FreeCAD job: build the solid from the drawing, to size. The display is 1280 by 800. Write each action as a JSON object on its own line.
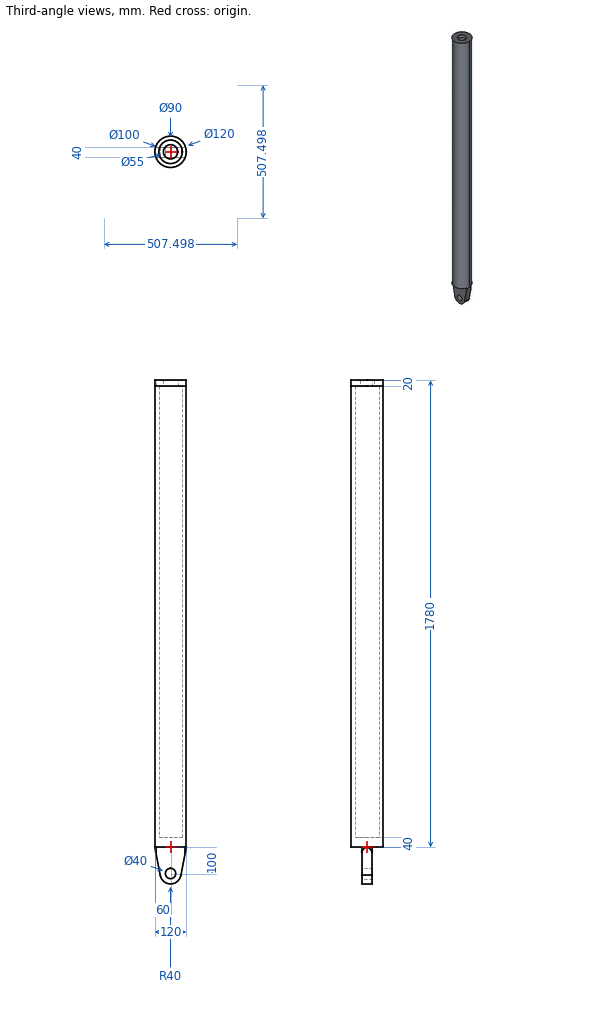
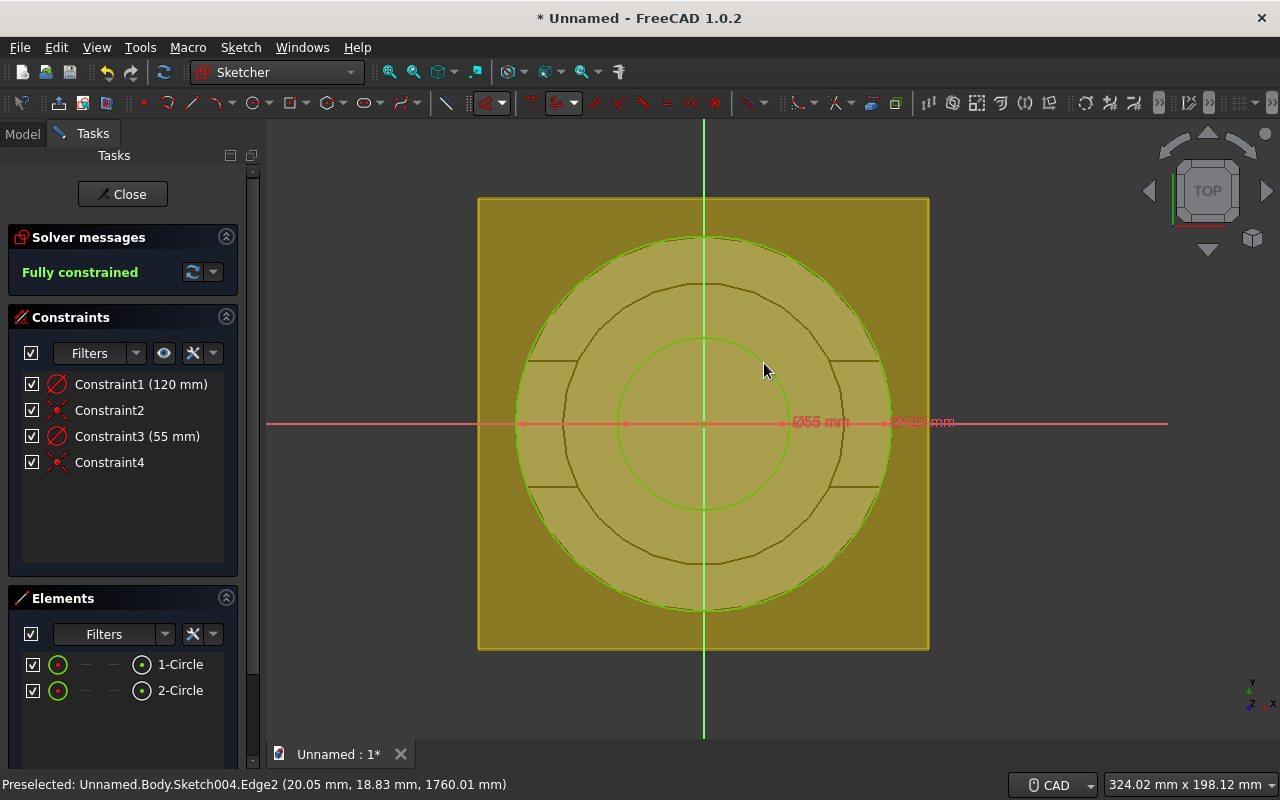
{"action": "left_click", "coordinate": [123, 194]}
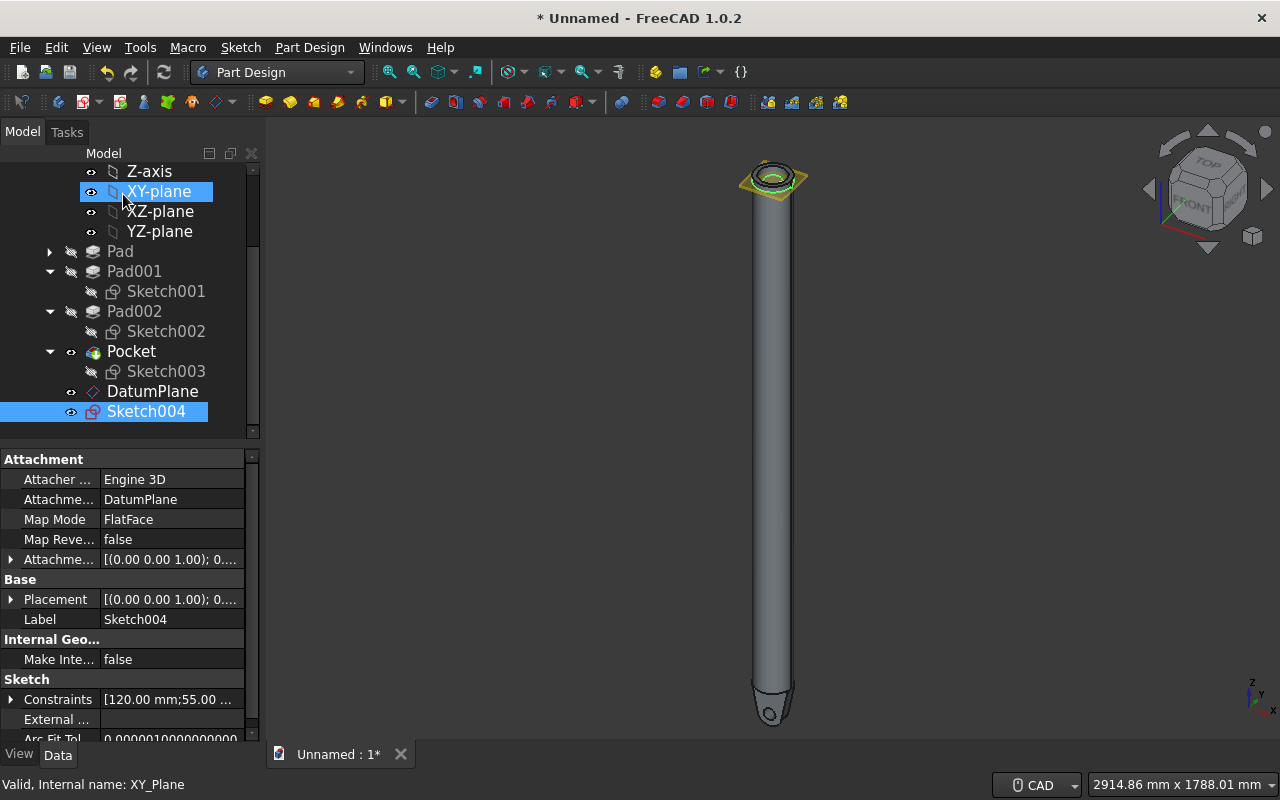
{"action": "left_click", "coordinate": [266, 102]}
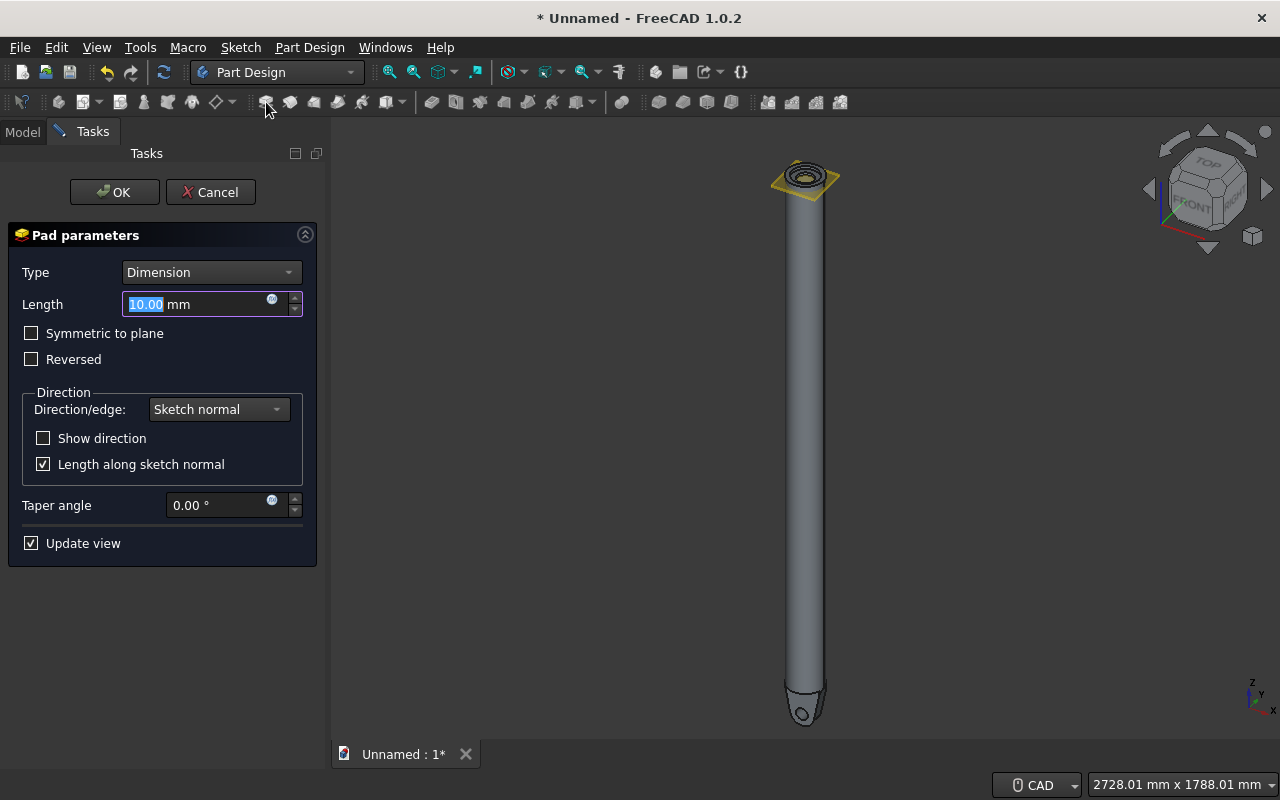
{"action": "type", "text": "20"}
{"action": "key", "text": "Tab"}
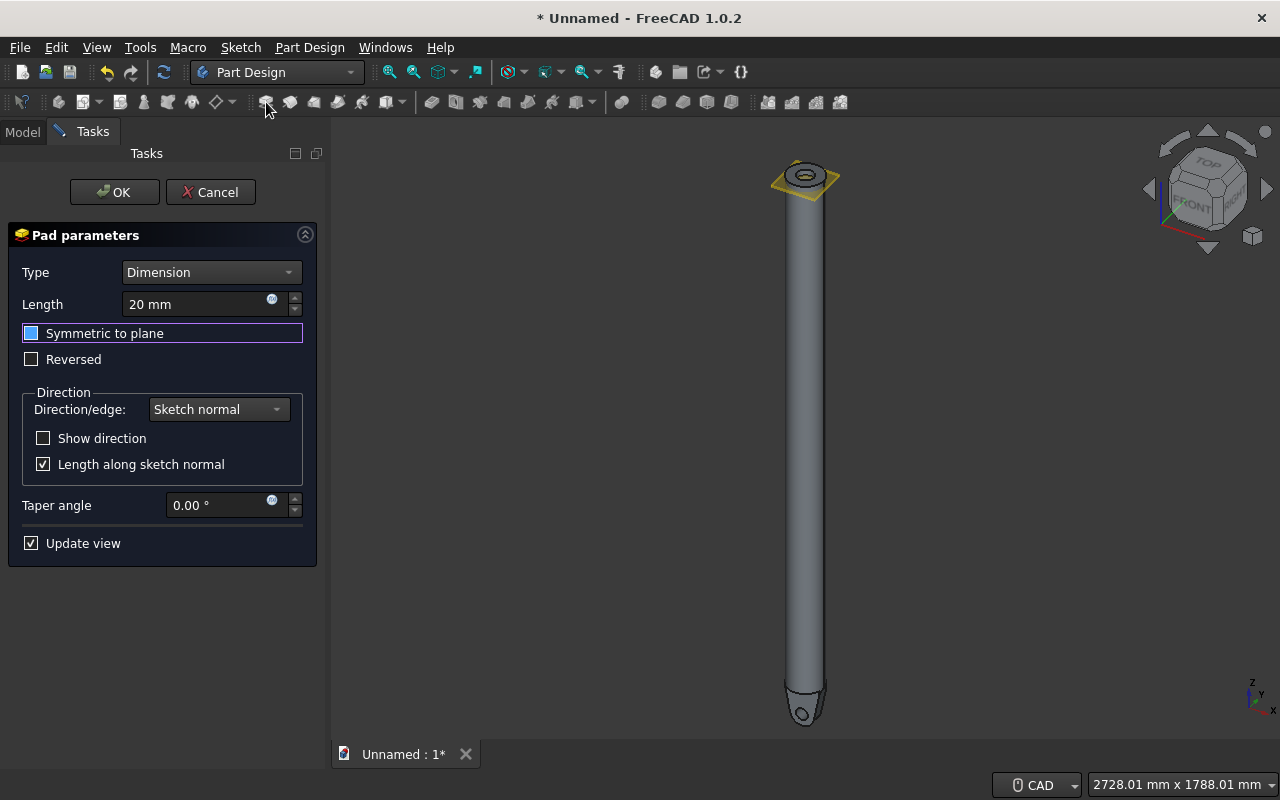
{"action": "left_click", "coordinate": [115, 192]}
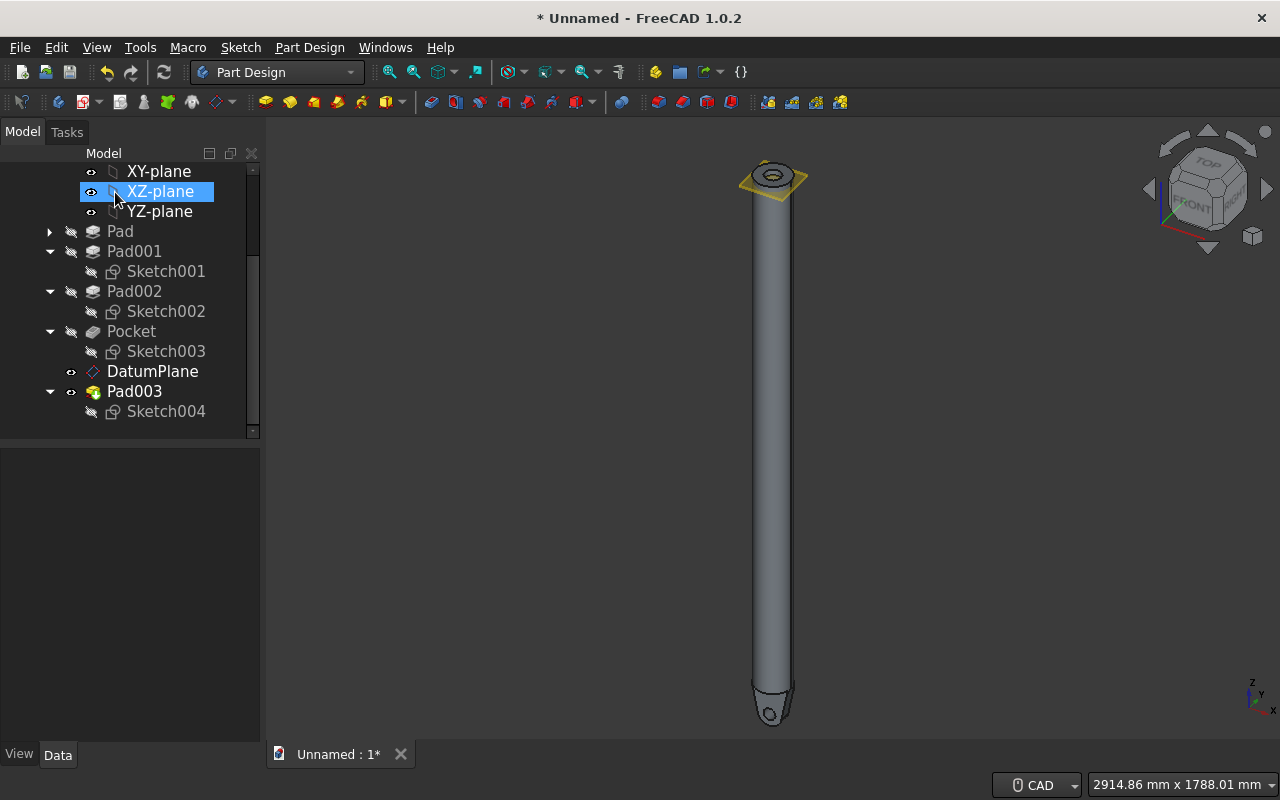
{"action": "left_click", "coordinate": [116, 372]}
{"action": "key", "text": "space"}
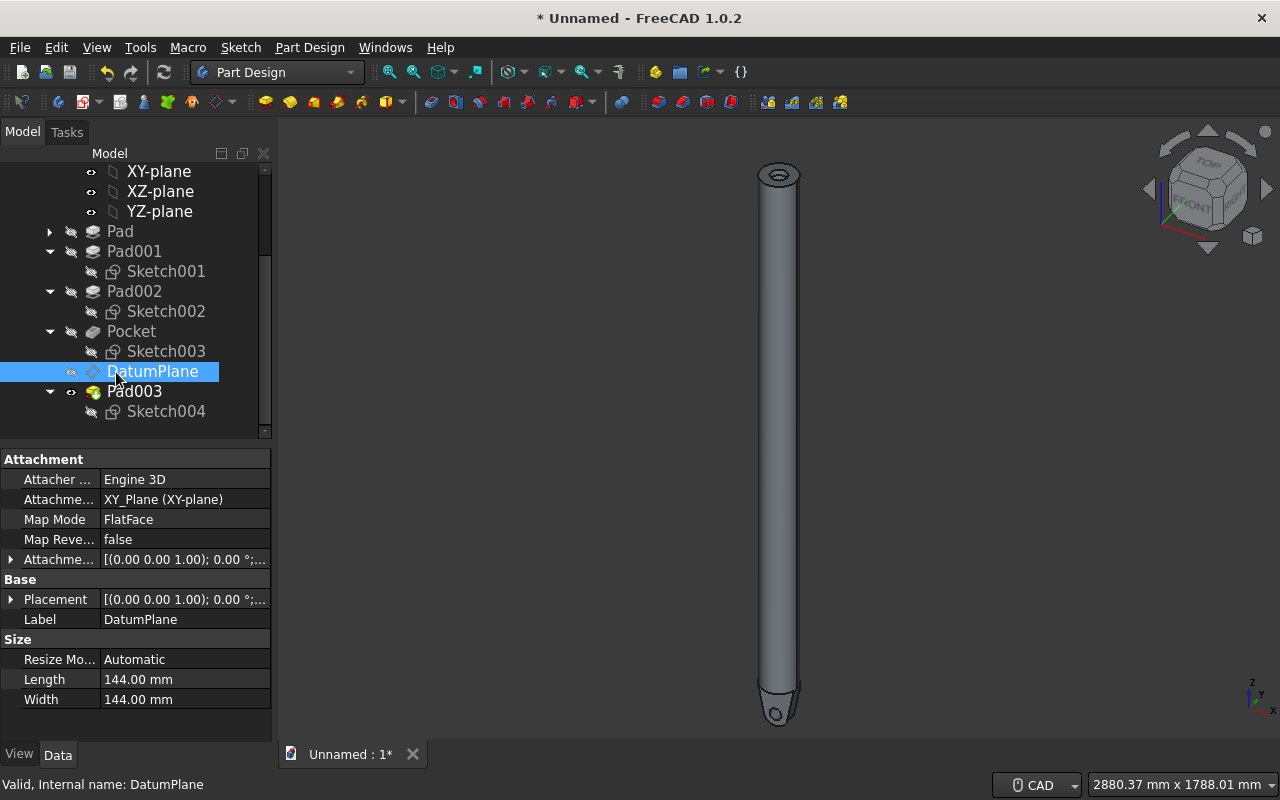
{"action": "key", "text": "0"}